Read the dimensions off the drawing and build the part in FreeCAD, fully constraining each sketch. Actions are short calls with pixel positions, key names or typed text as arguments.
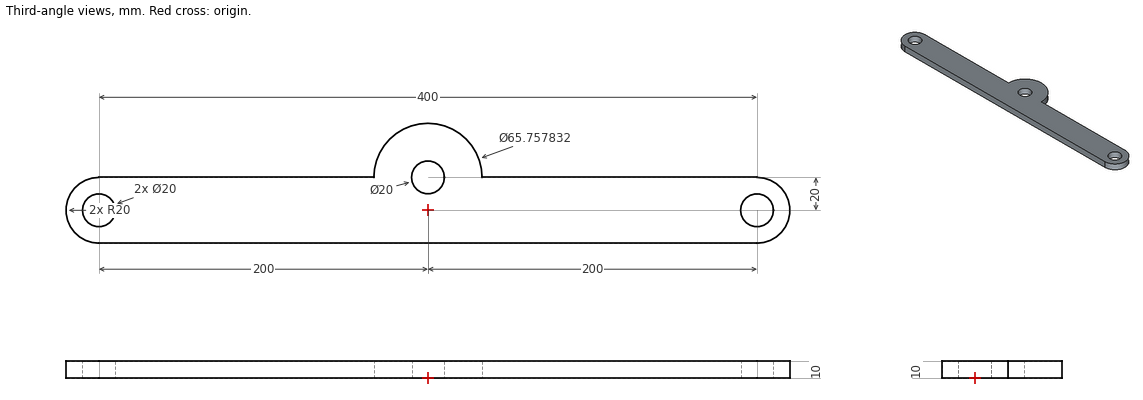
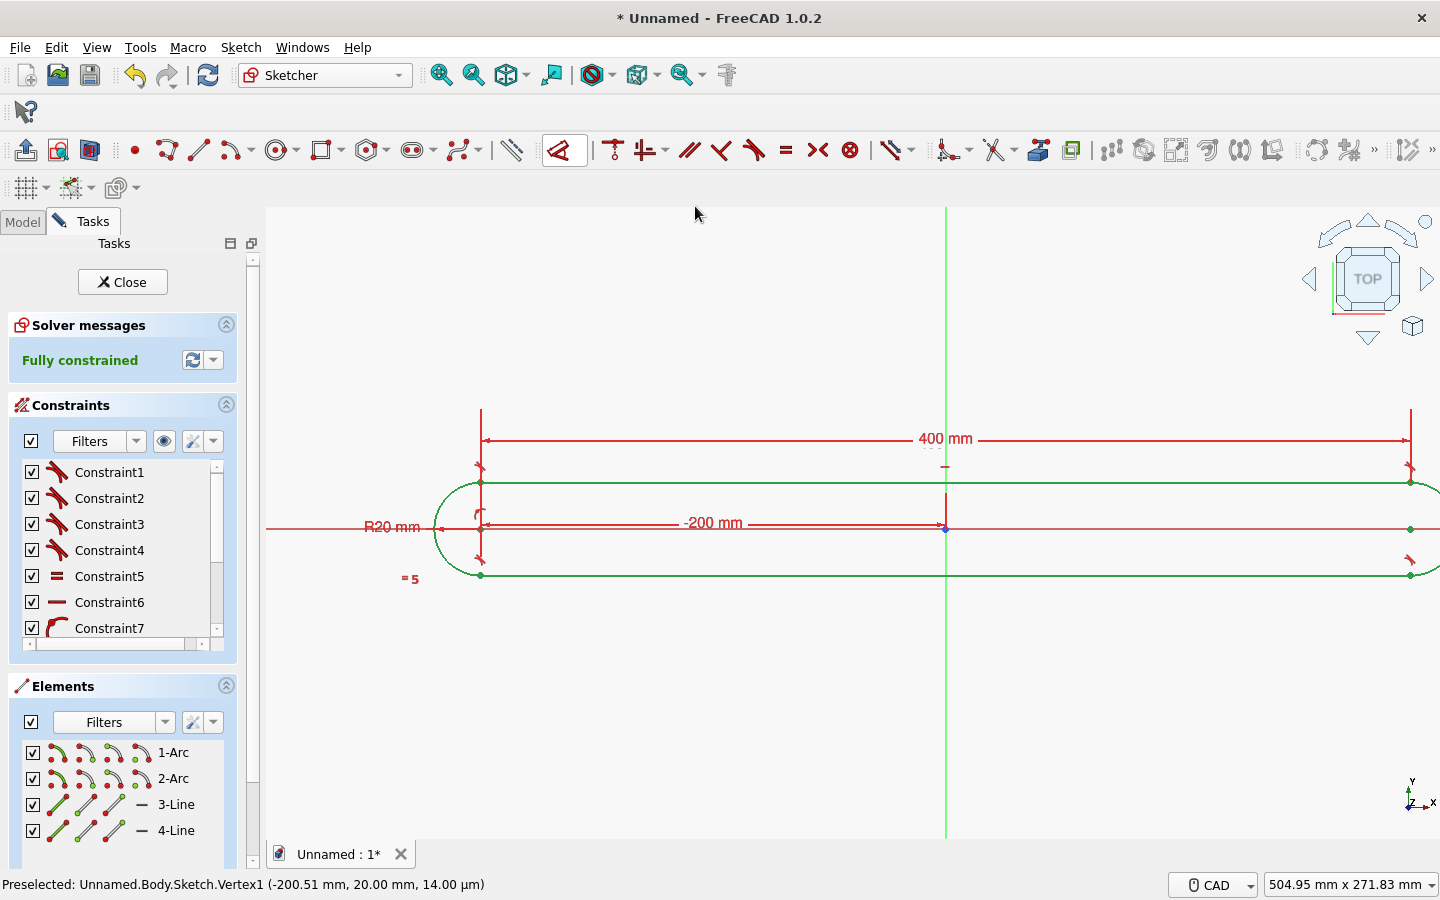
click(123, 282)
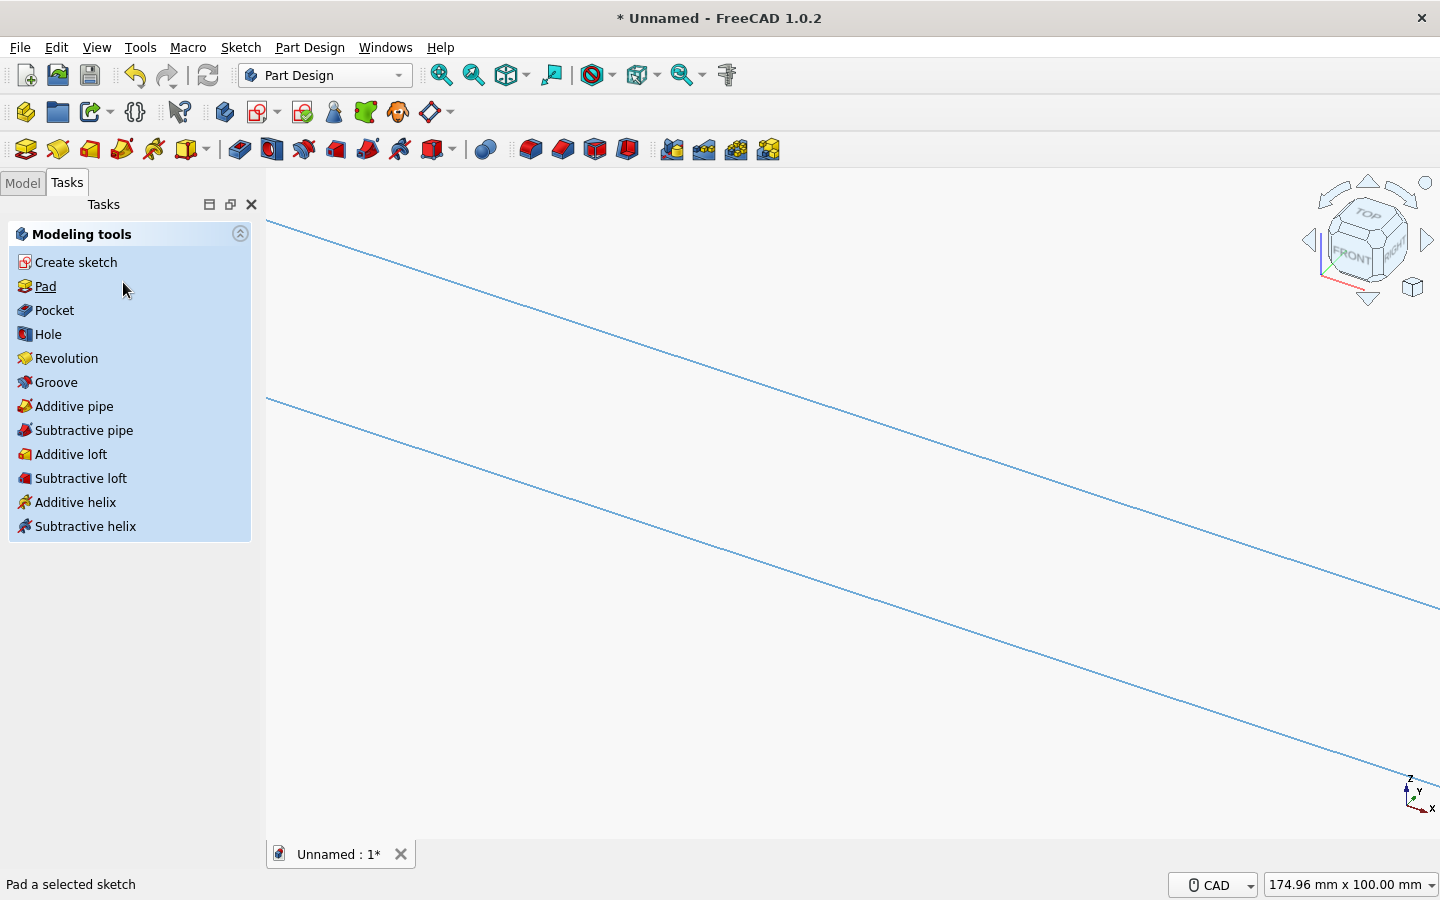
click(26, 150)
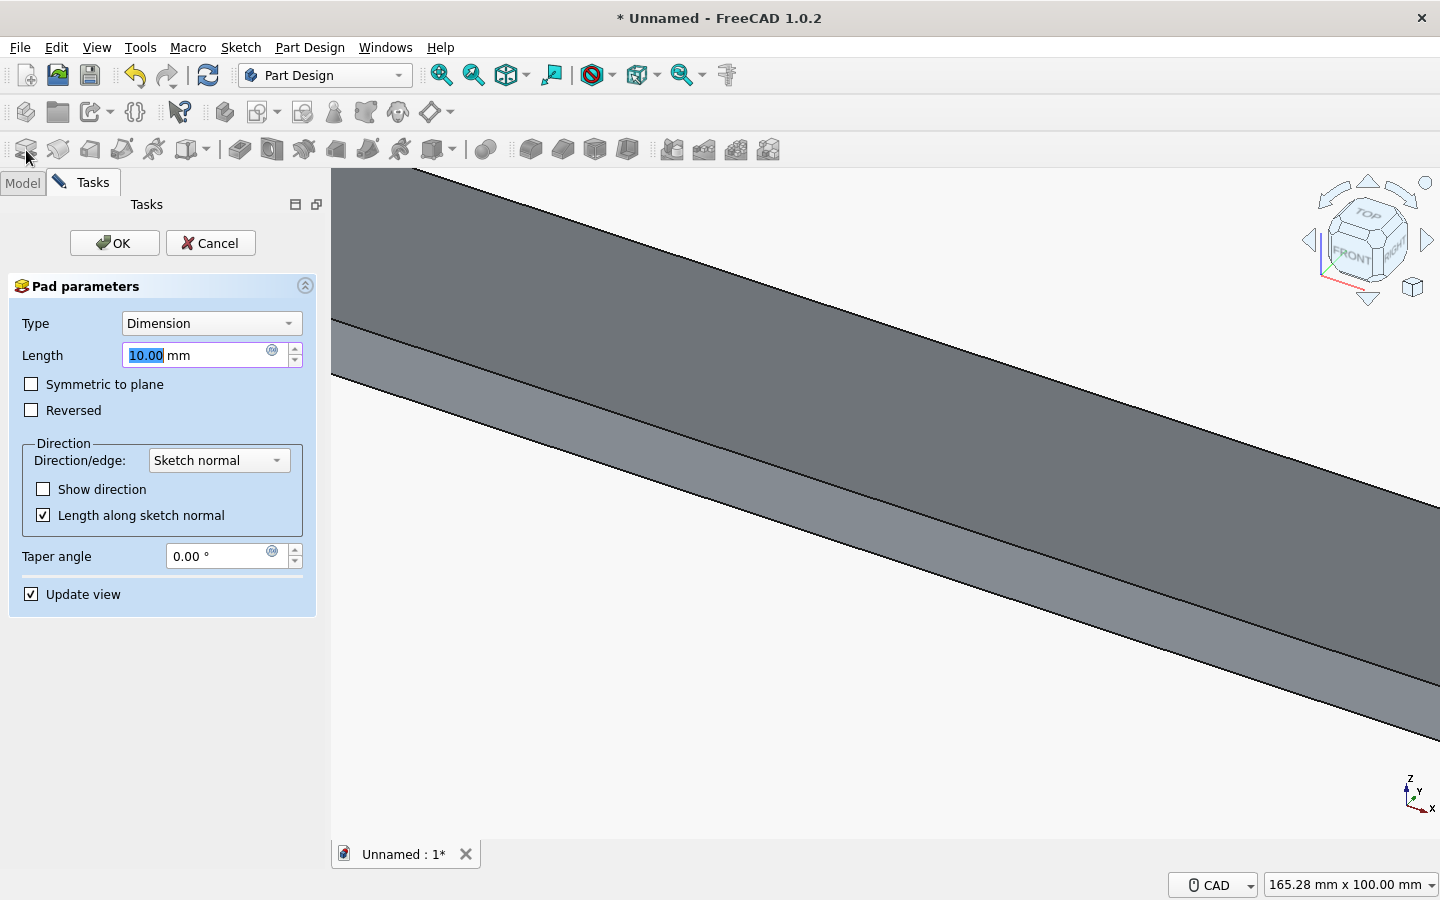
text(10)
key(Tab)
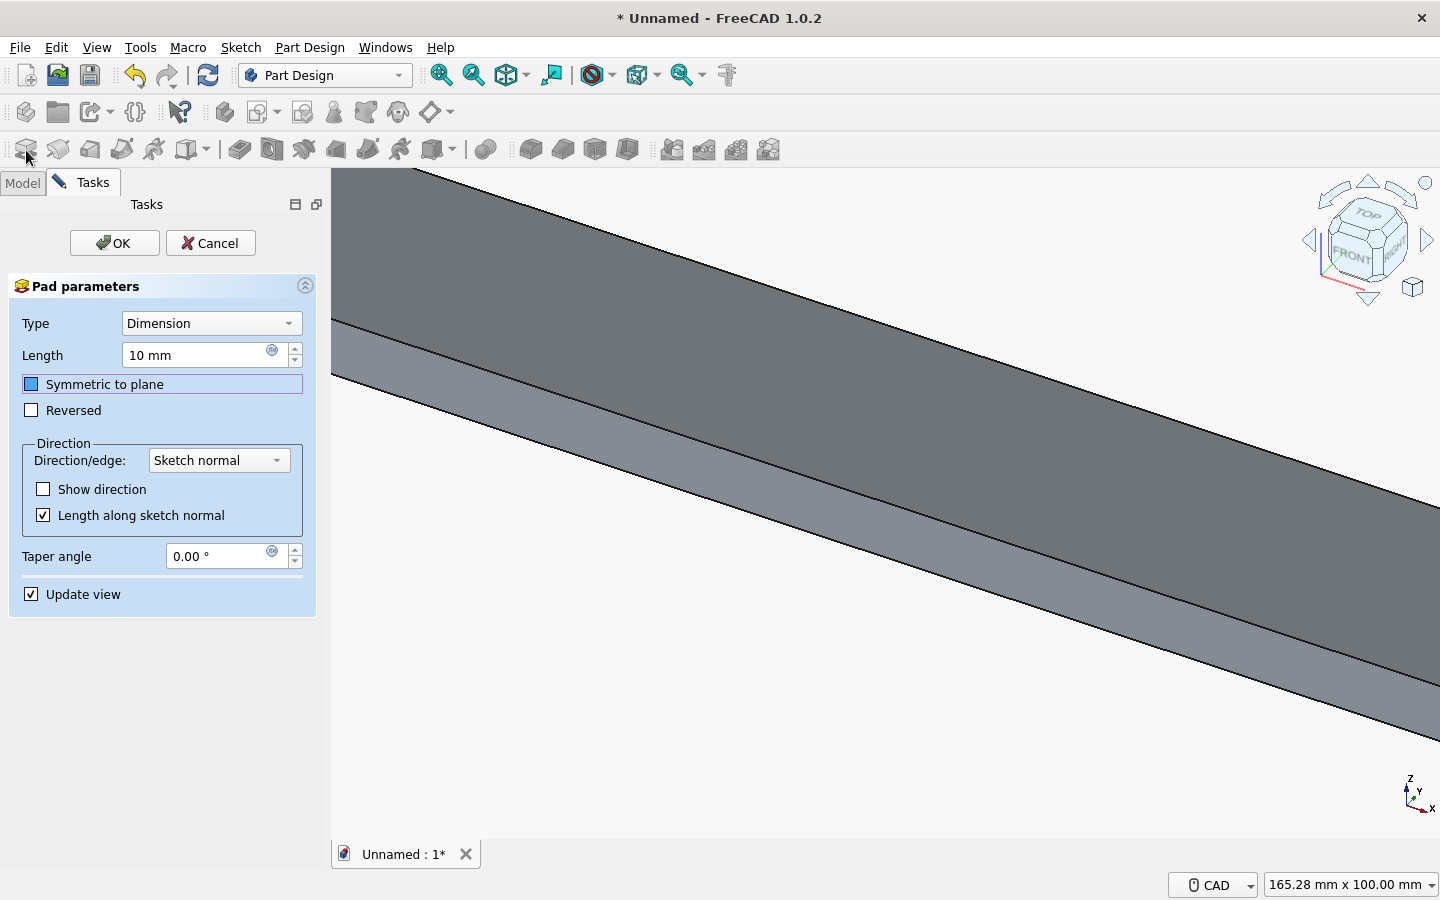
click(115, 243)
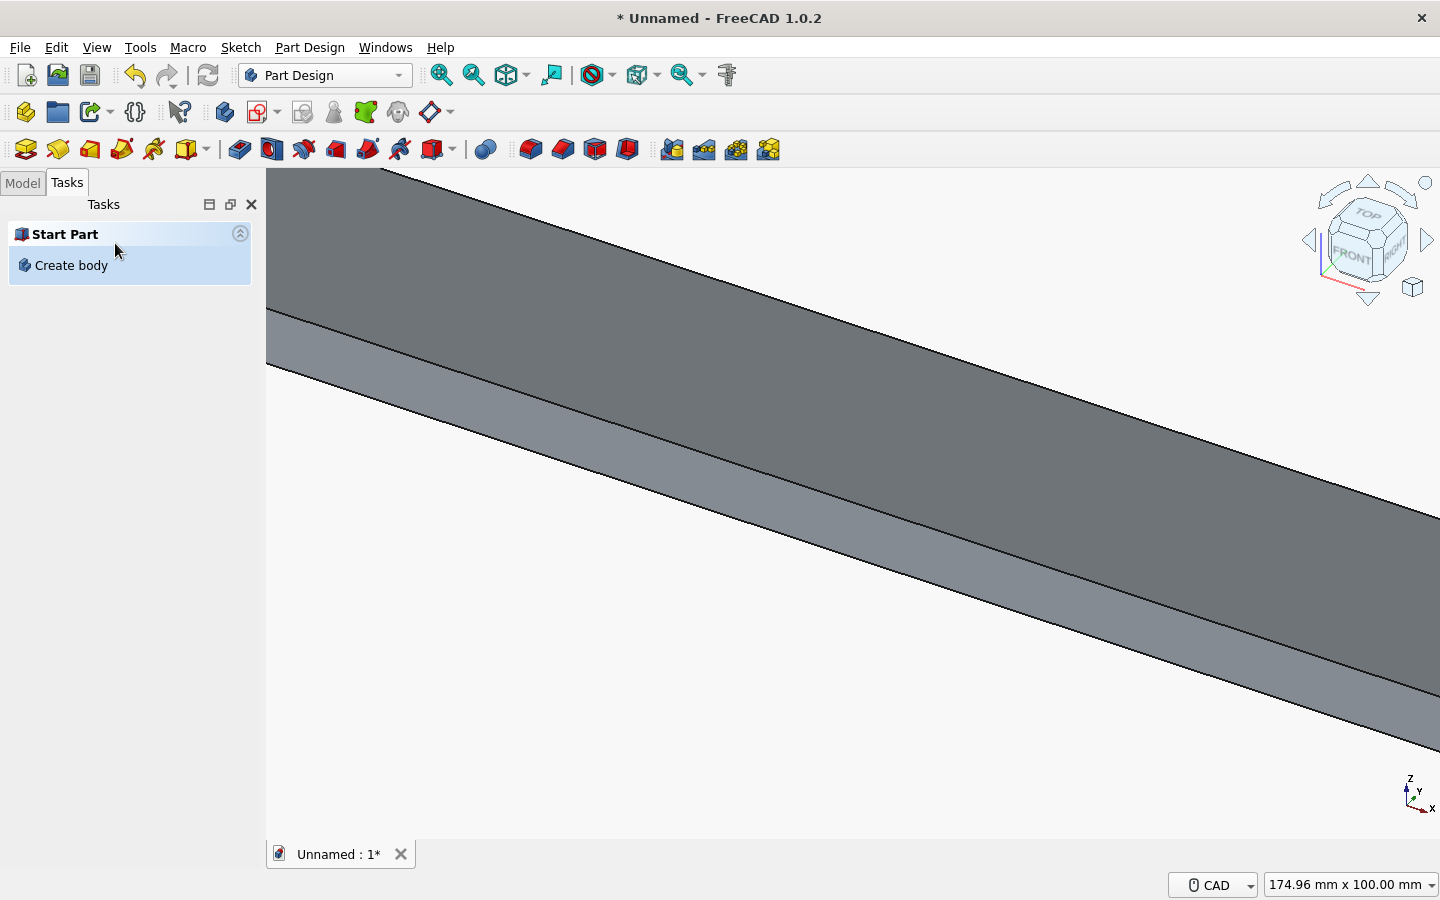
click(442, 76)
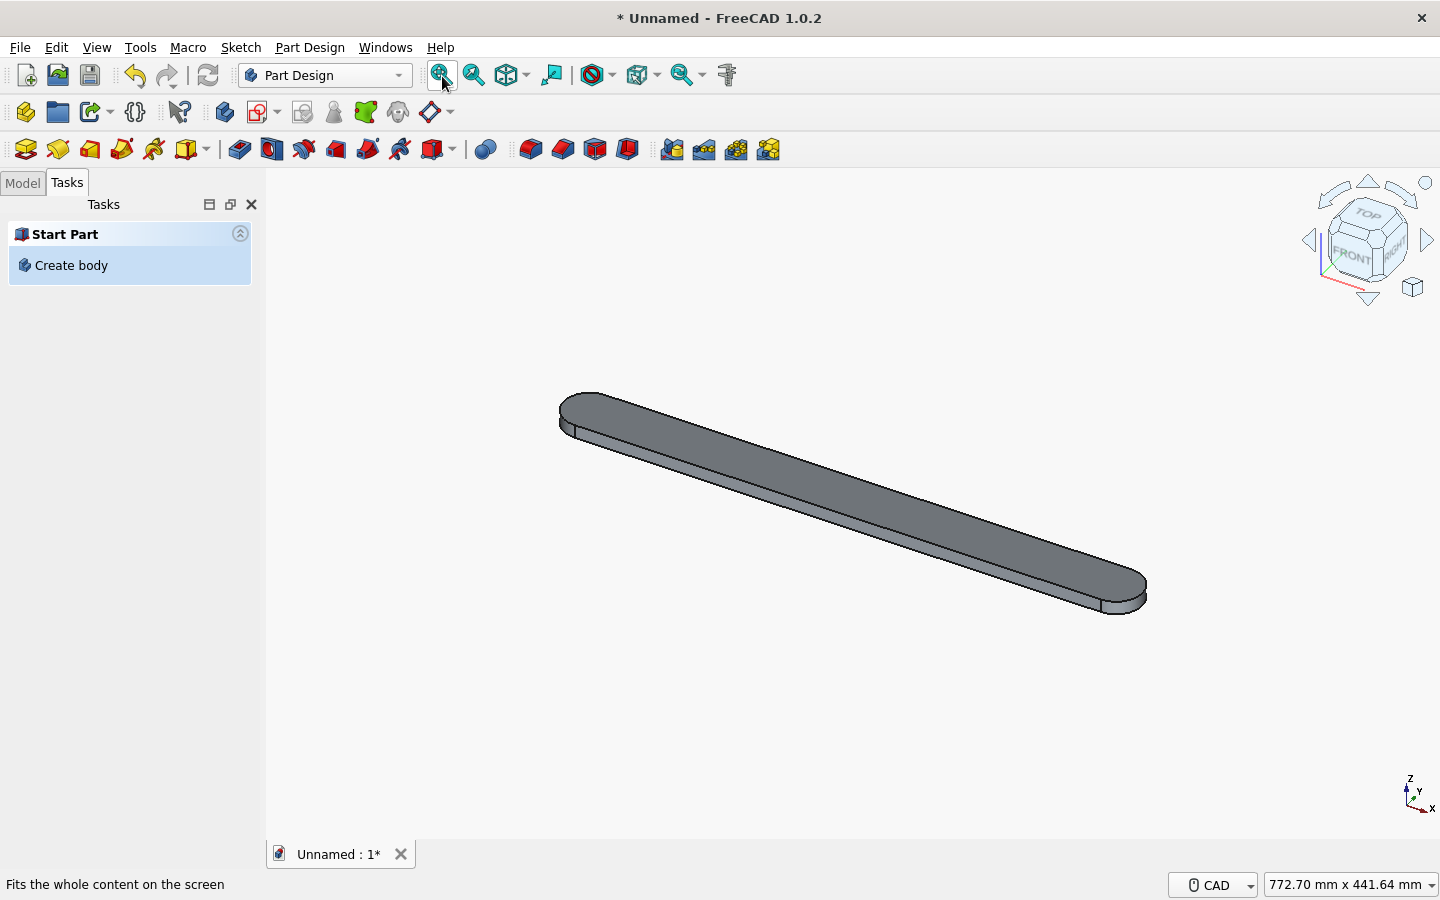
click(1101, 578)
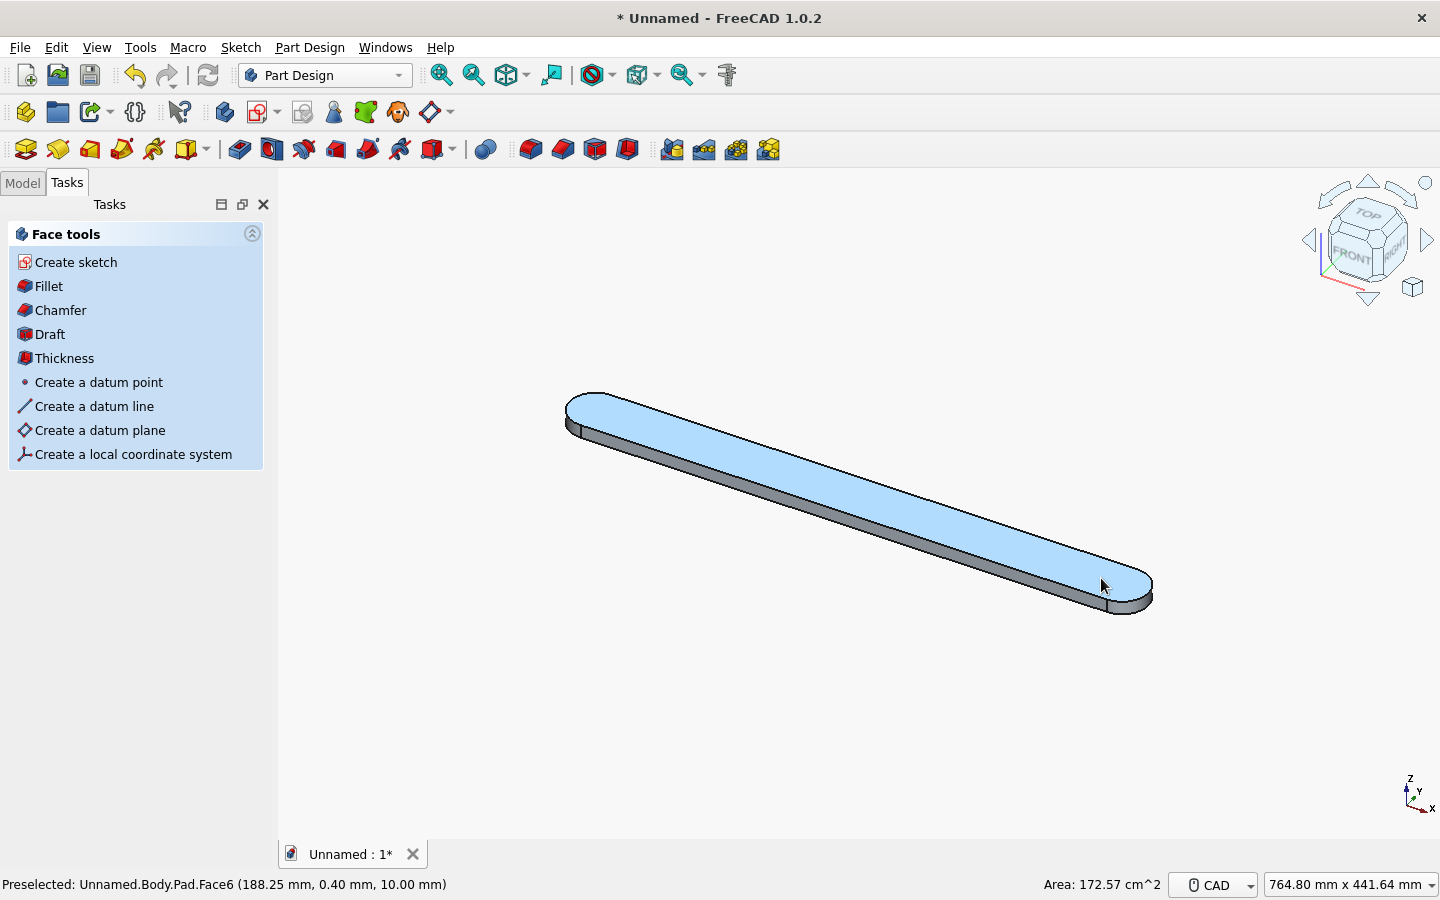
click(258, 112)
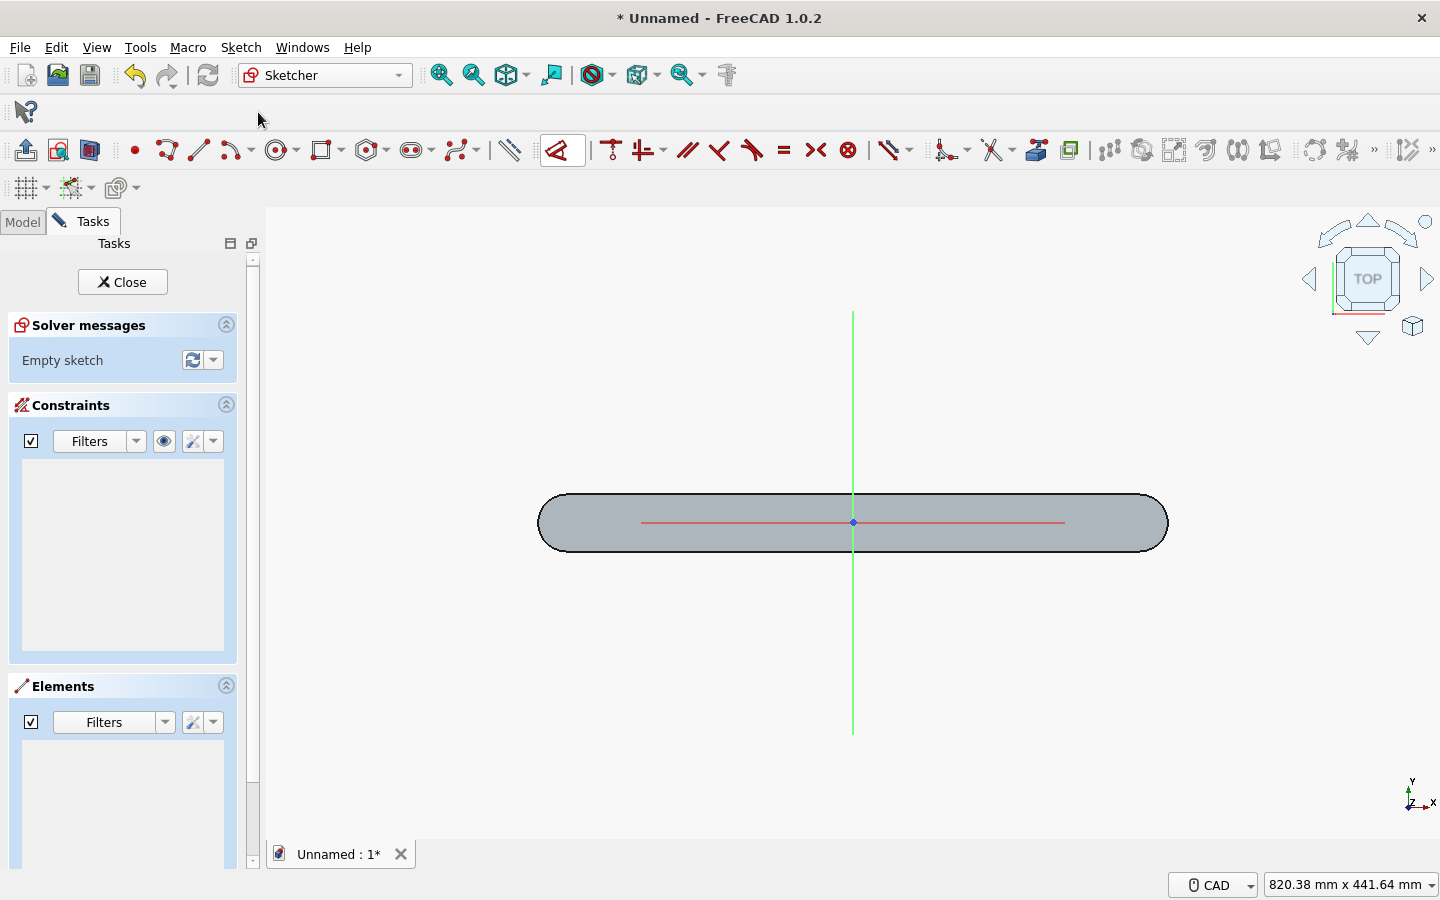
click(276, 150)